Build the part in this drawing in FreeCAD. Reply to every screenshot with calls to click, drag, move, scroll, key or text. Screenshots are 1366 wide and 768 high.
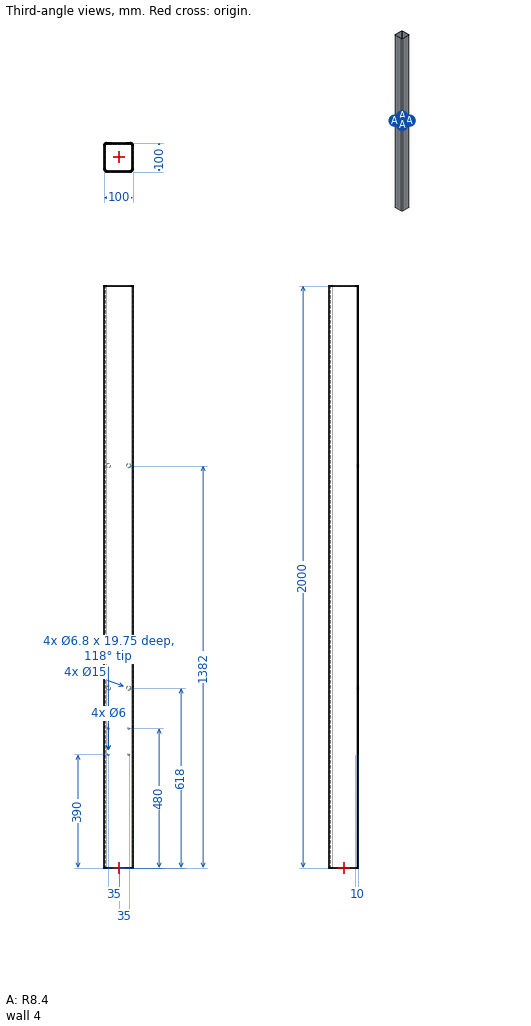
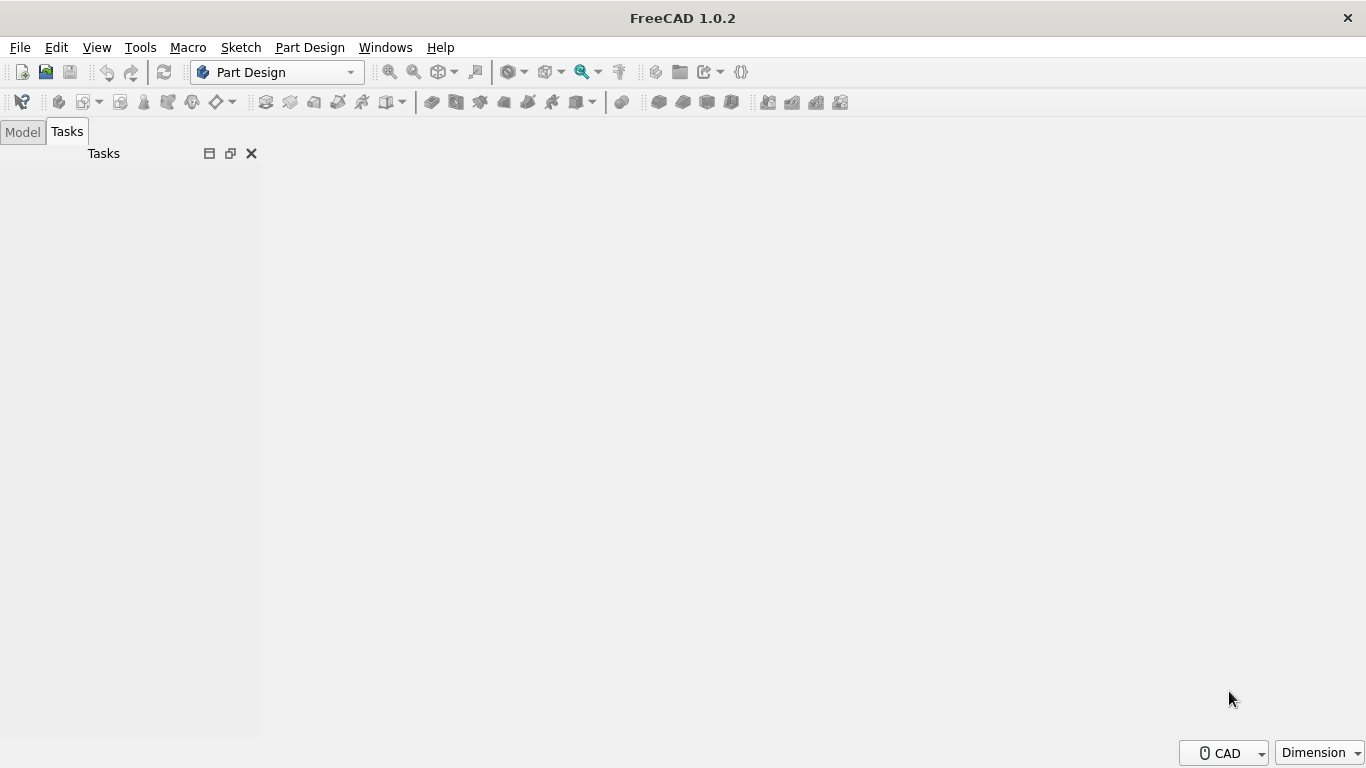
click(22, 72)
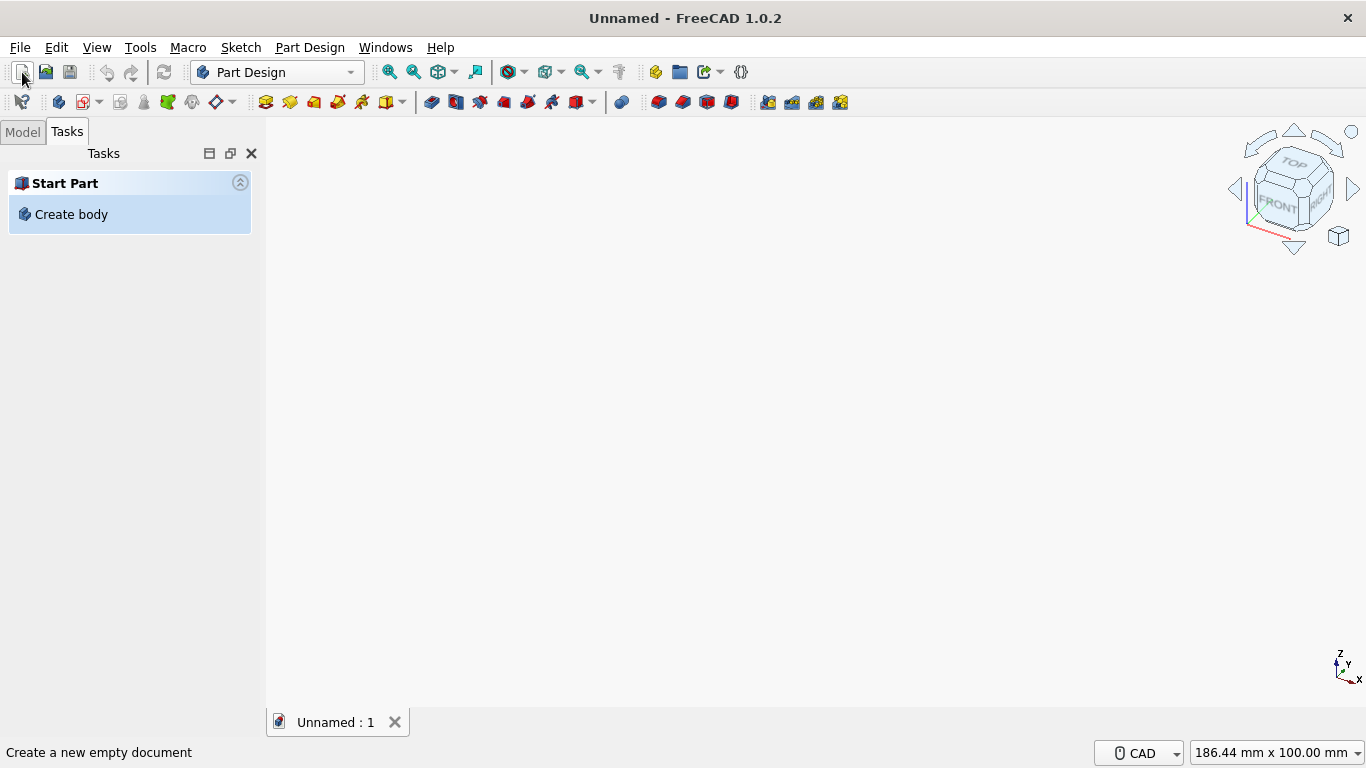
click(84, 102)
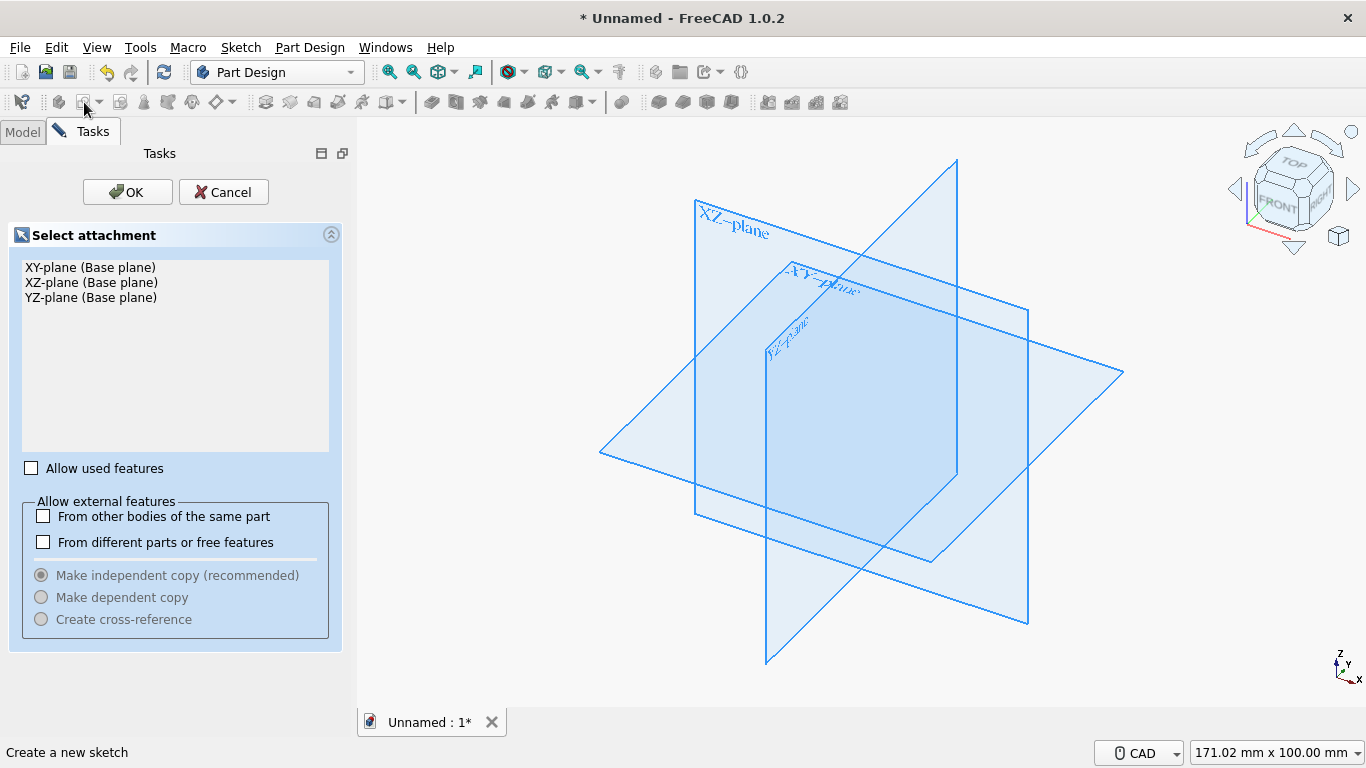
click(82, 268)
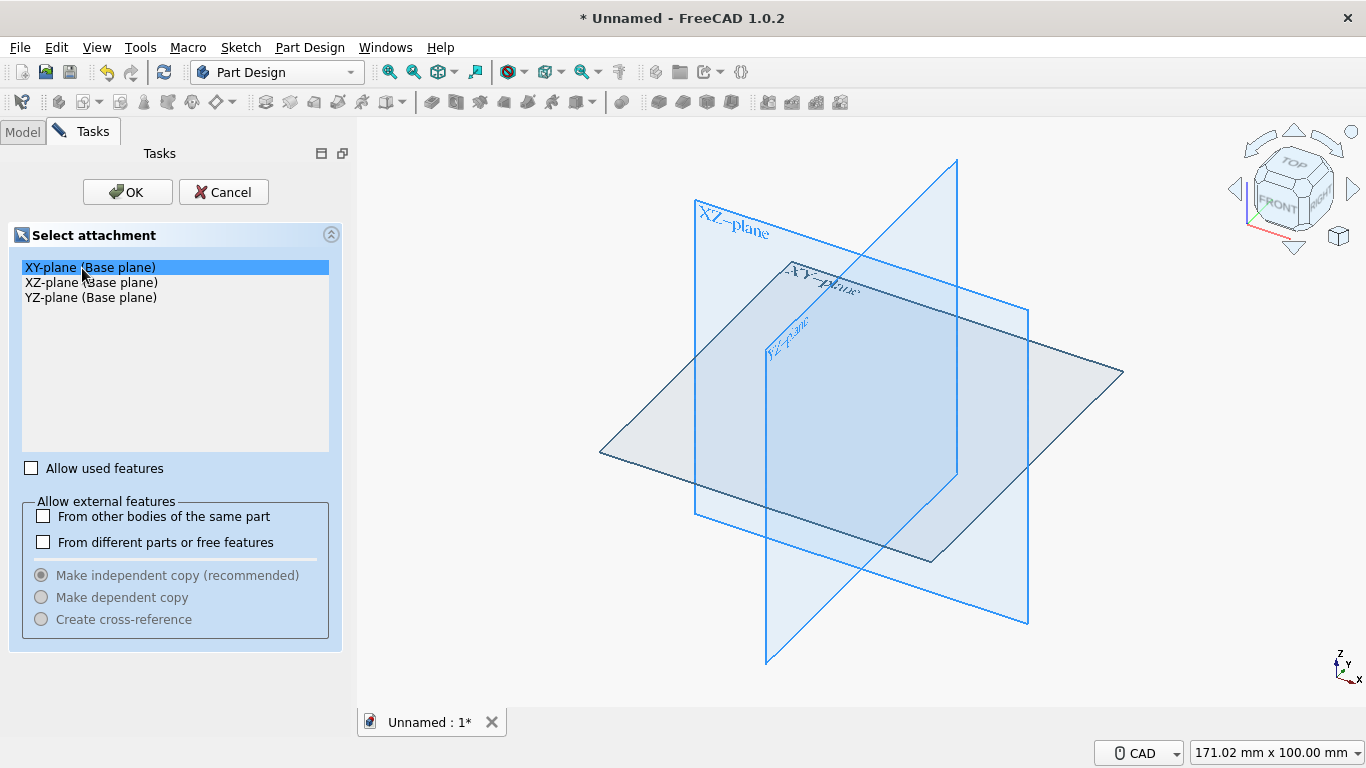
click(128, 192)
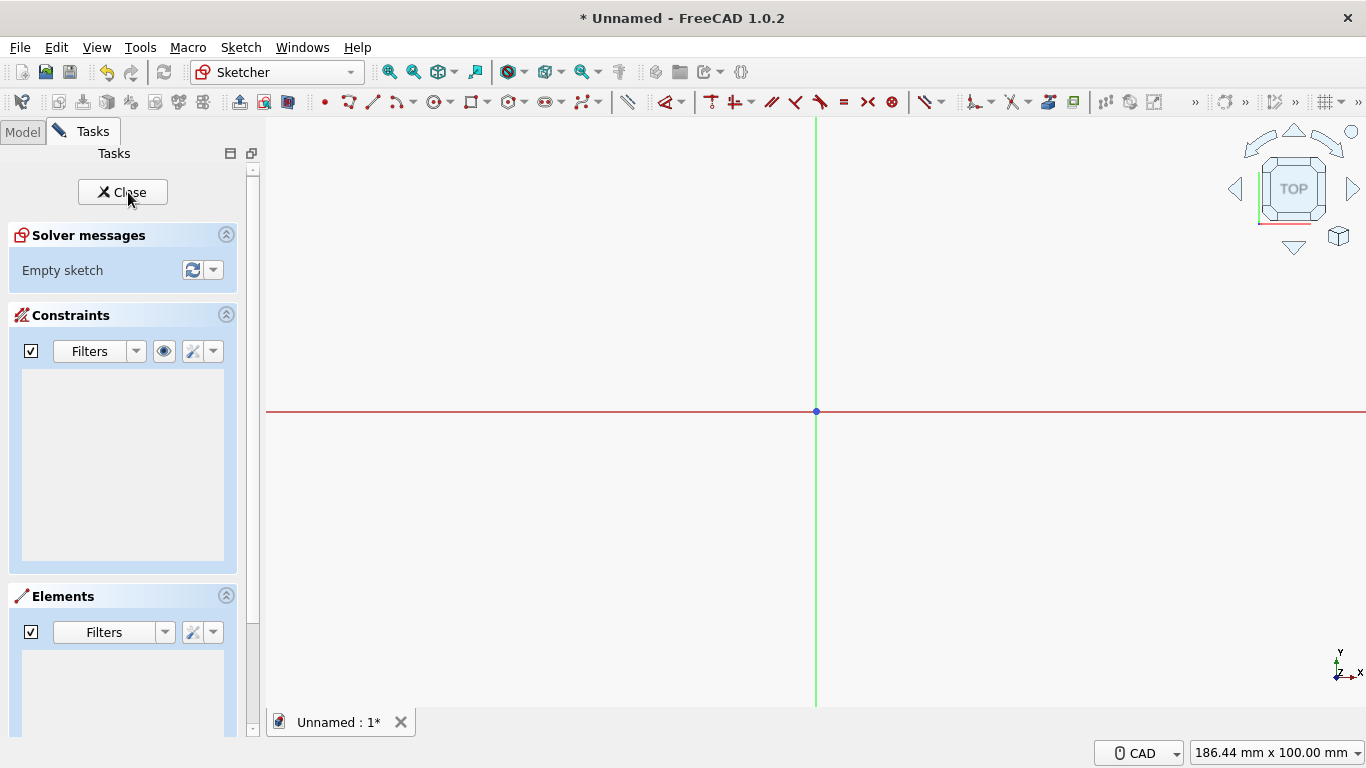
scroll(608, 412, down, 2)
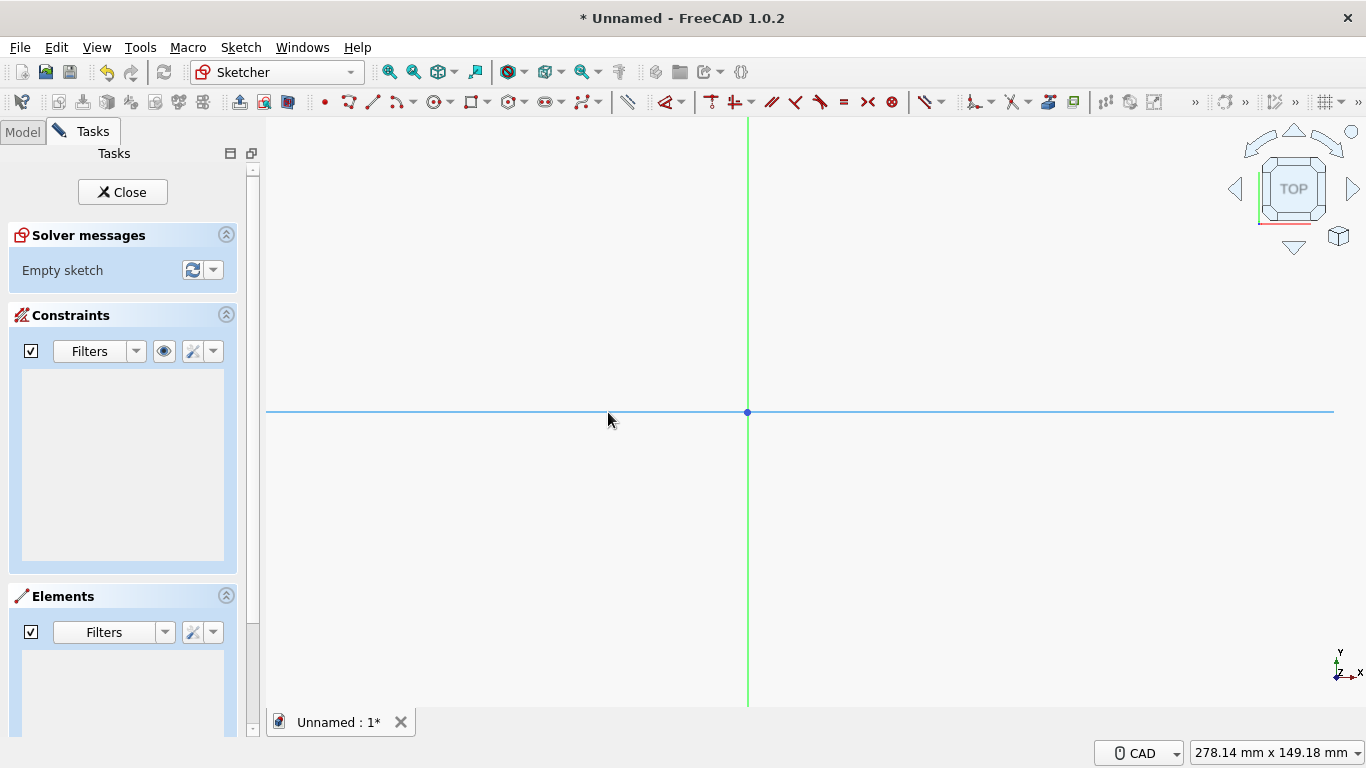
click(490, 102)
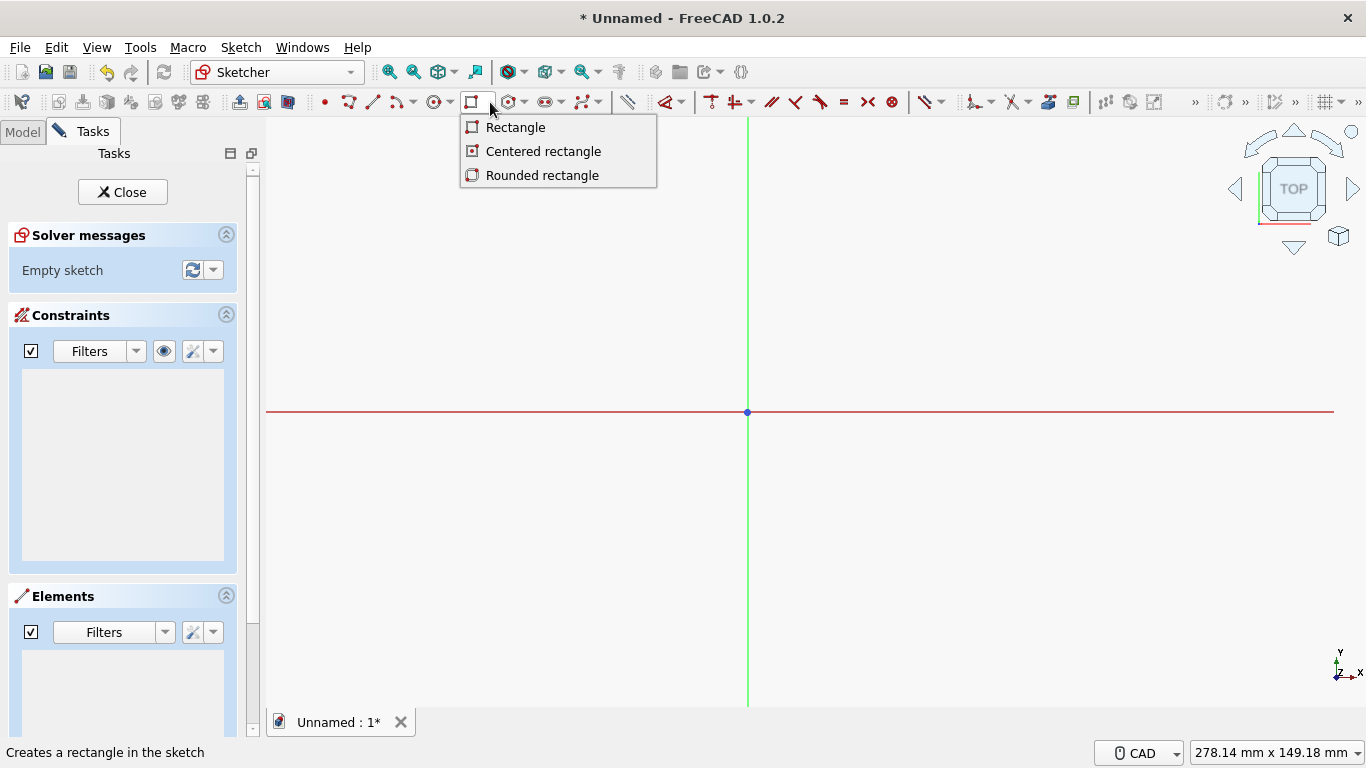
click(558, 151)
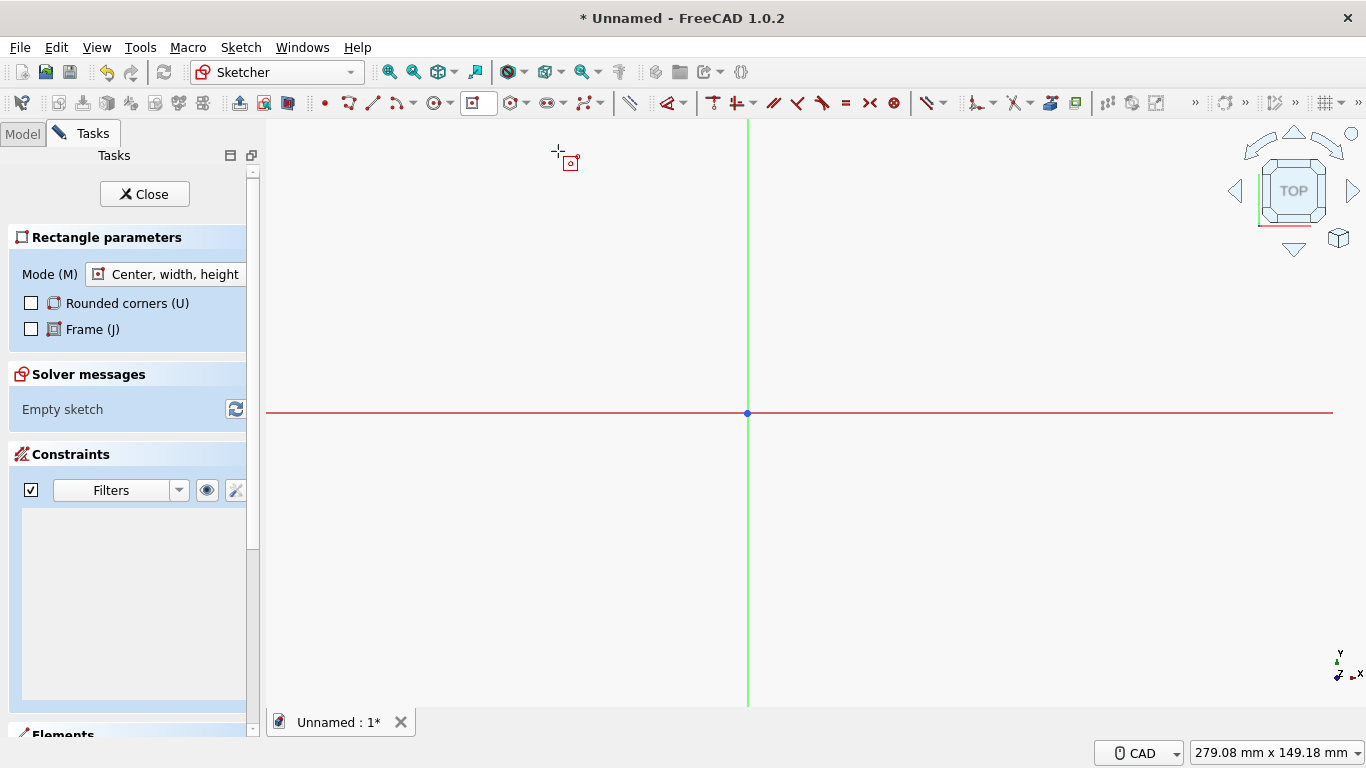
click(748, 413)
click(945, 216)
key(Escape)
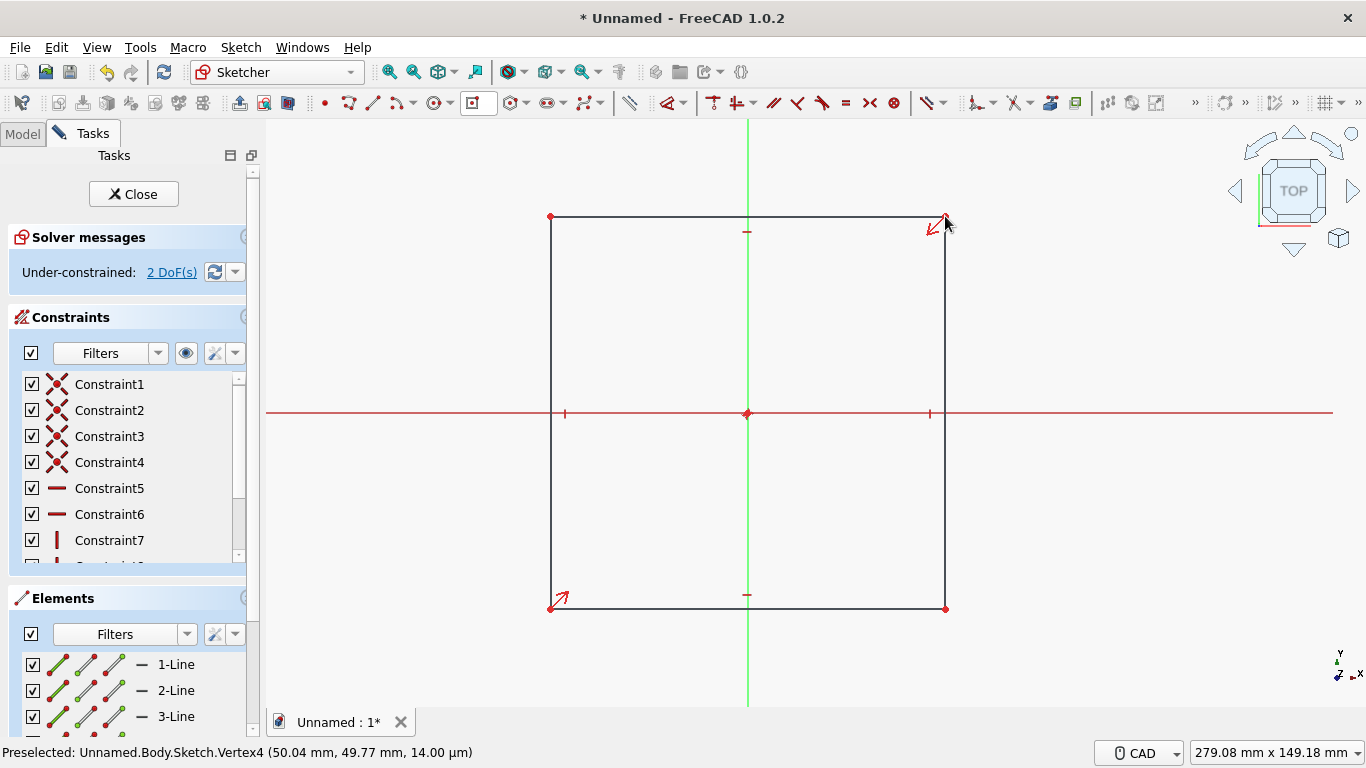
click(668, 104)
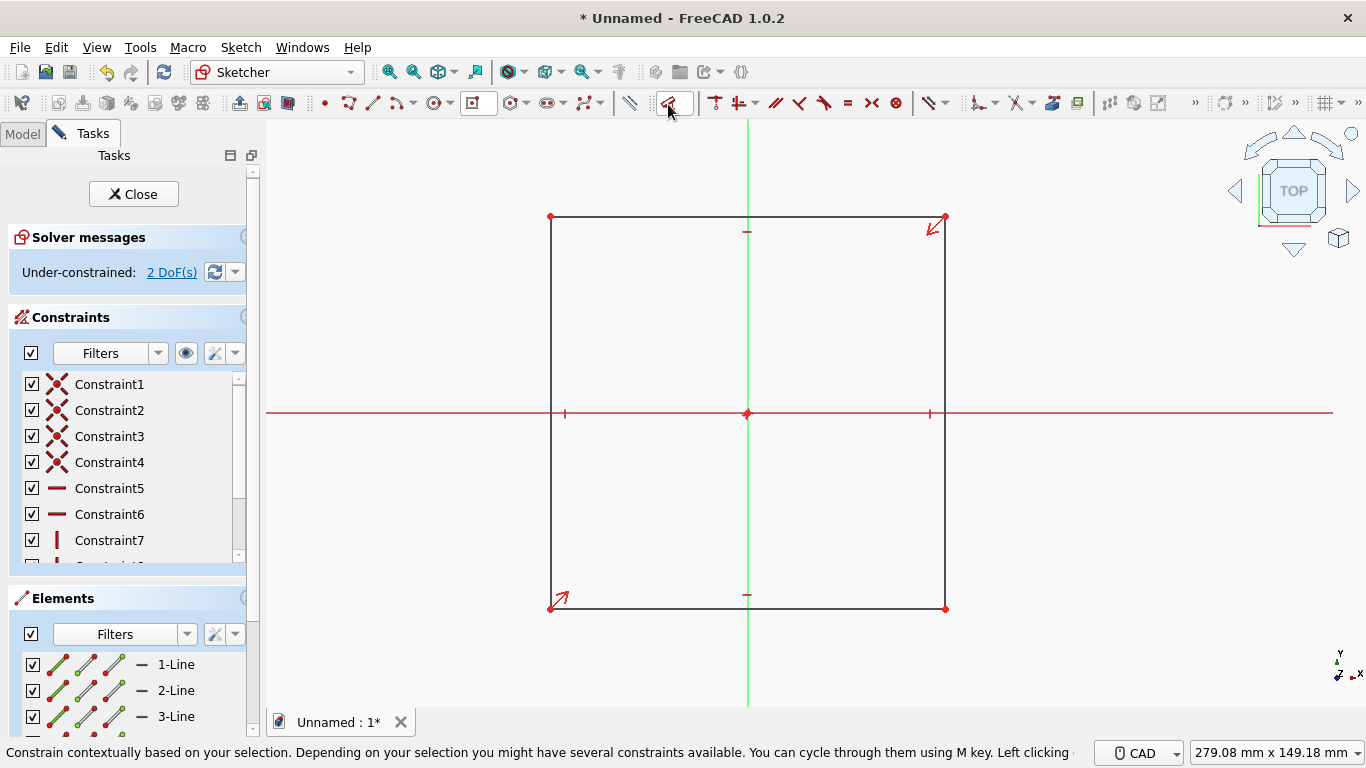
click(669, 609)
click(657, 643)